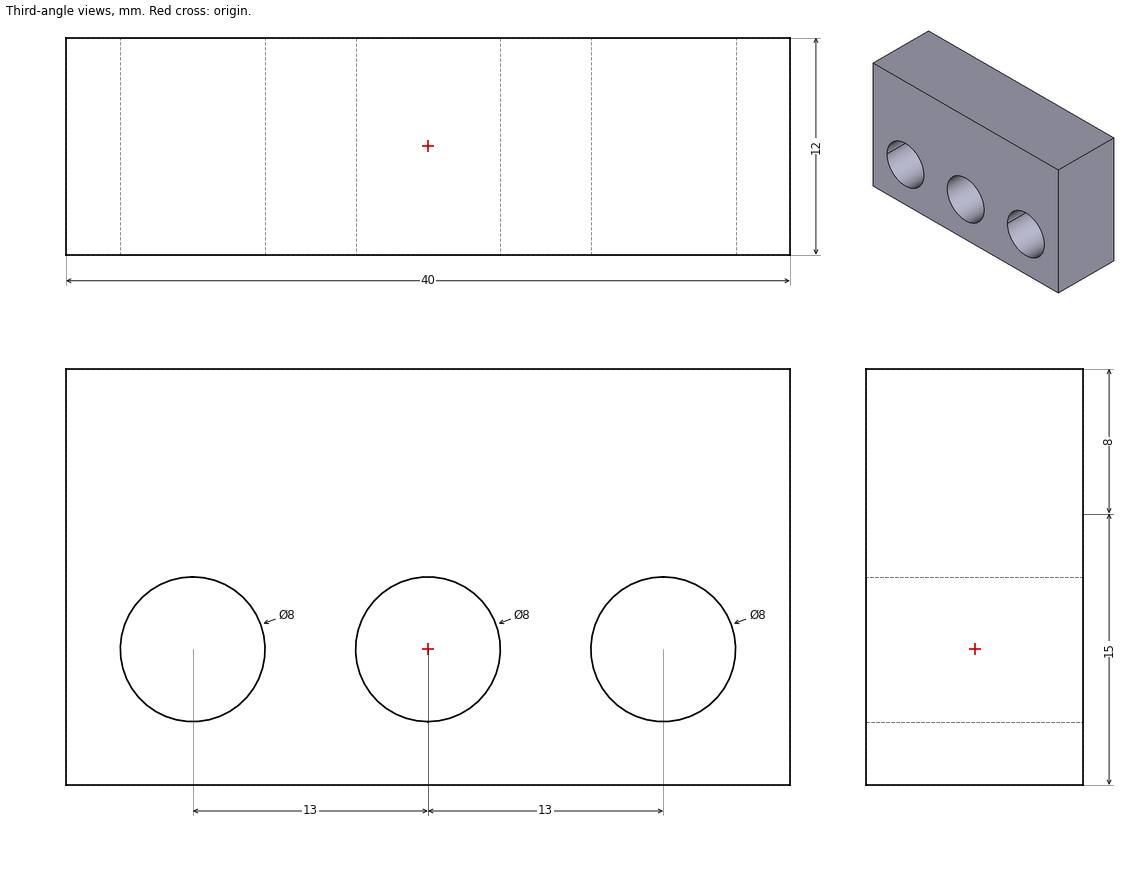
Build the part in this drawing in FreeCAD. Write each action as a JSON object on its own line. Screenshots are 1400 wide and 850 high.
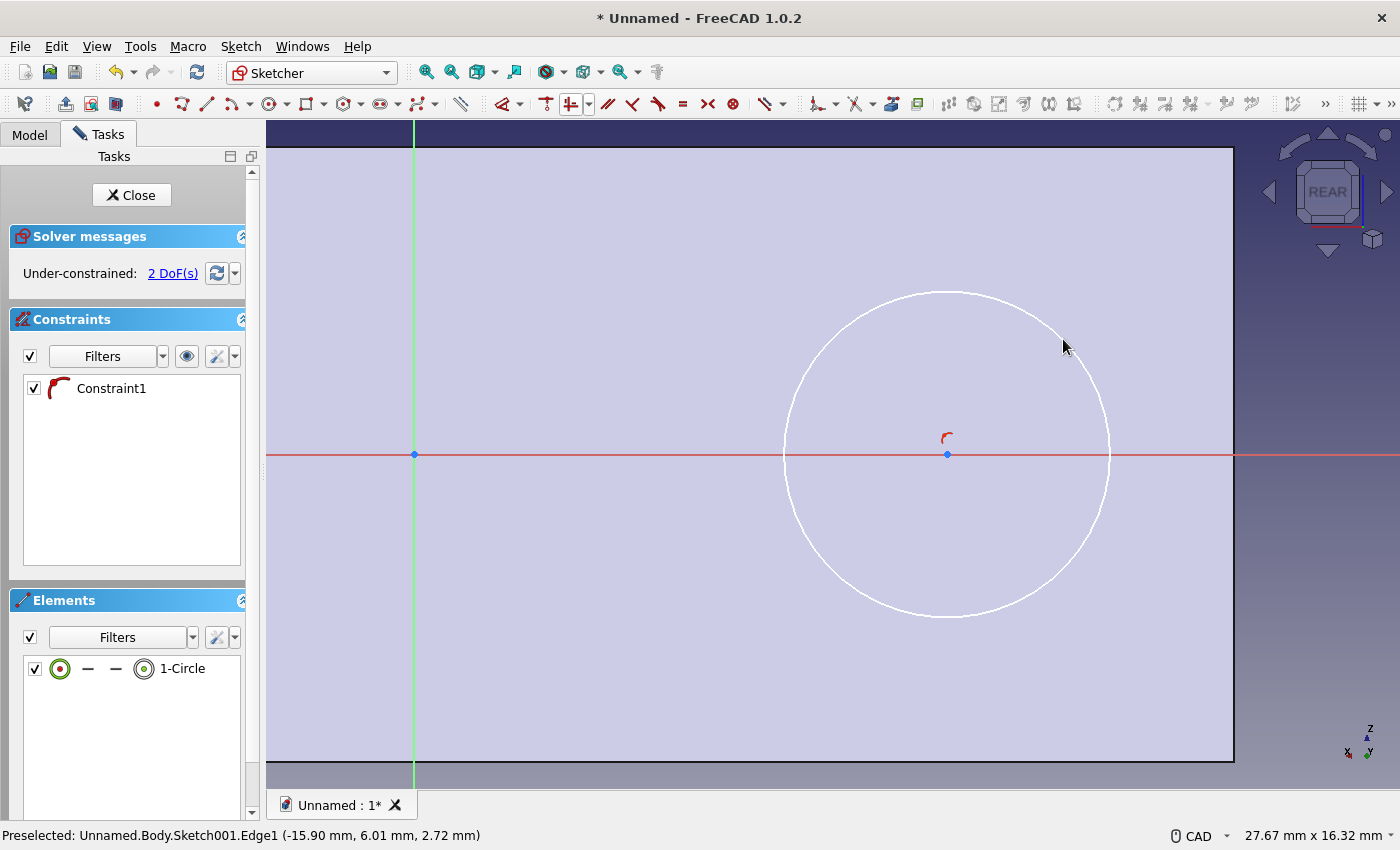
{"action": "key", "text": "d"}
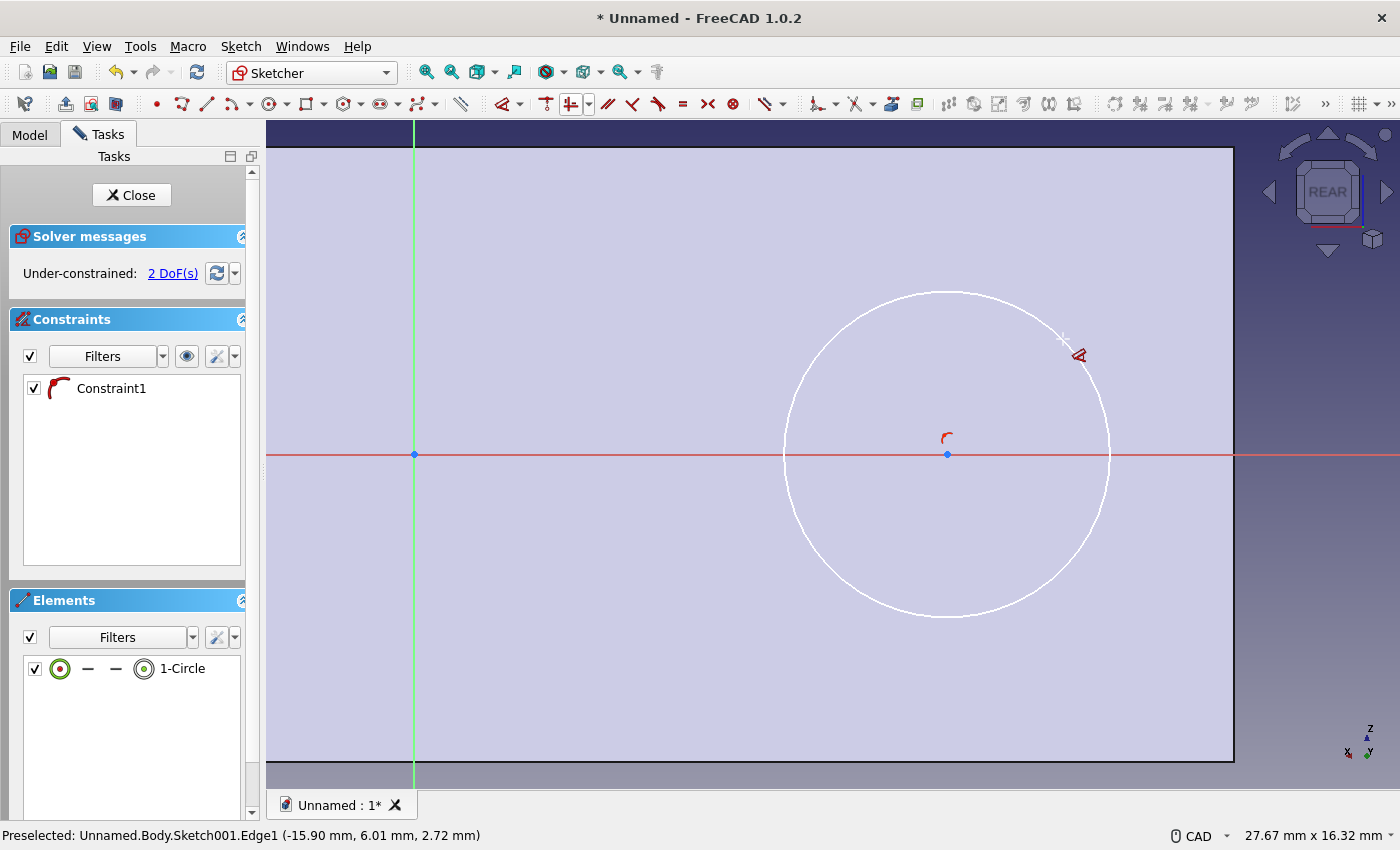
{"action": "left_click", "coordinate": [1062, 339]}
{"action": "left_click", "coordinate": [1085, 316]}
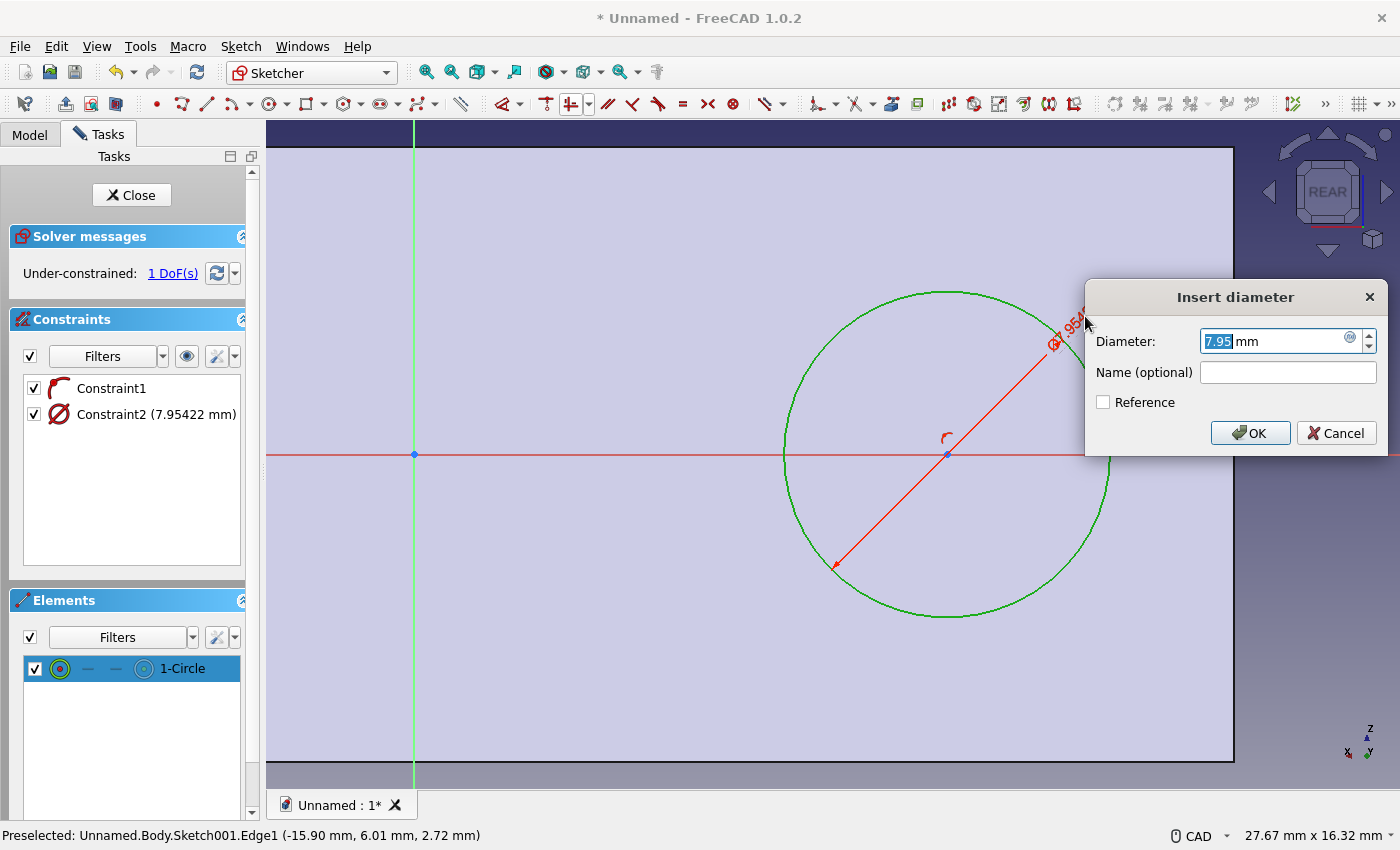
{"action": "type", "text": "8"}
{"action": "key", "text": "Return"}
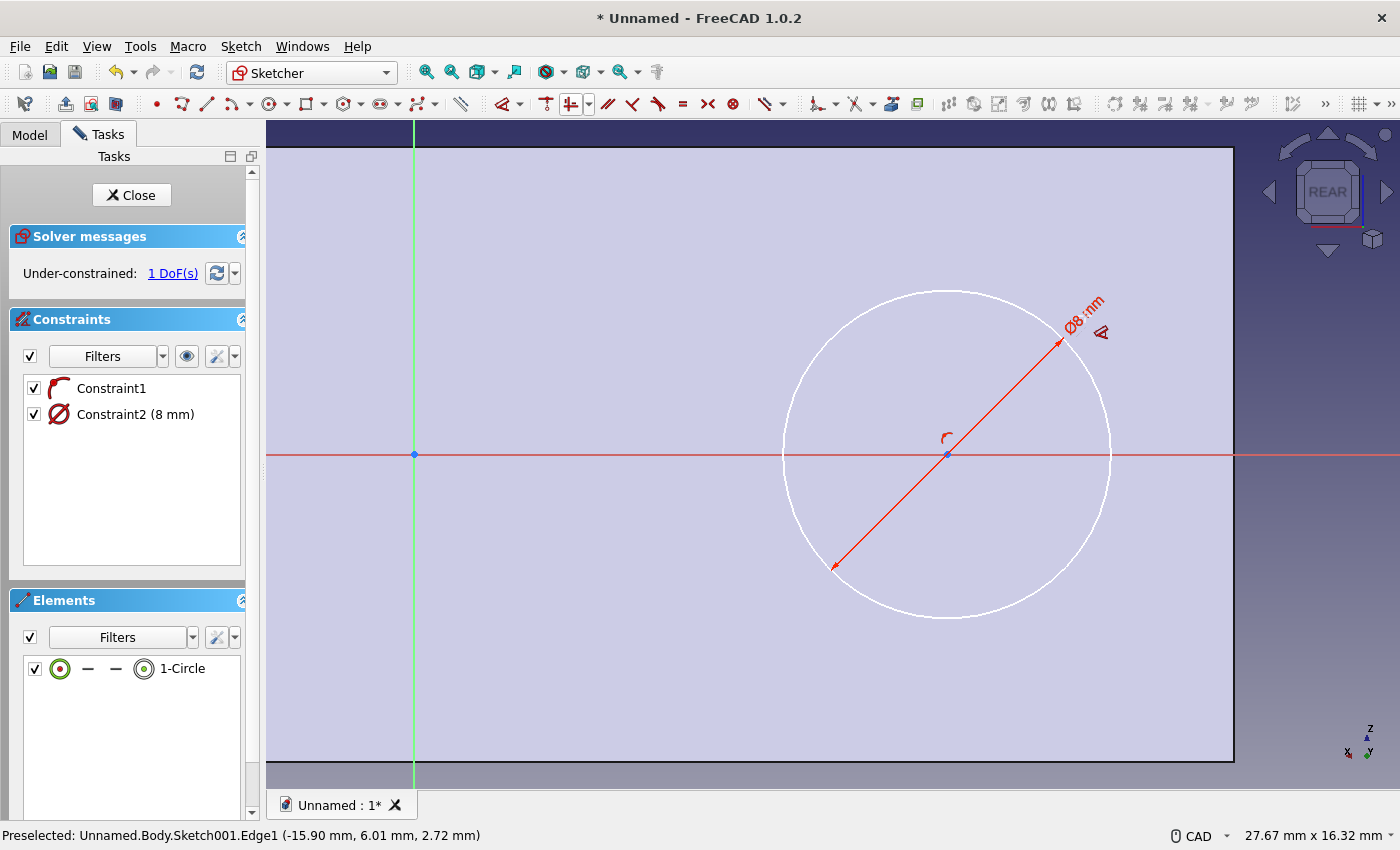
{"action": "left_click", "coordinate": [947, 454]}
{"action": "left_click", "coordinate": [681, 488]}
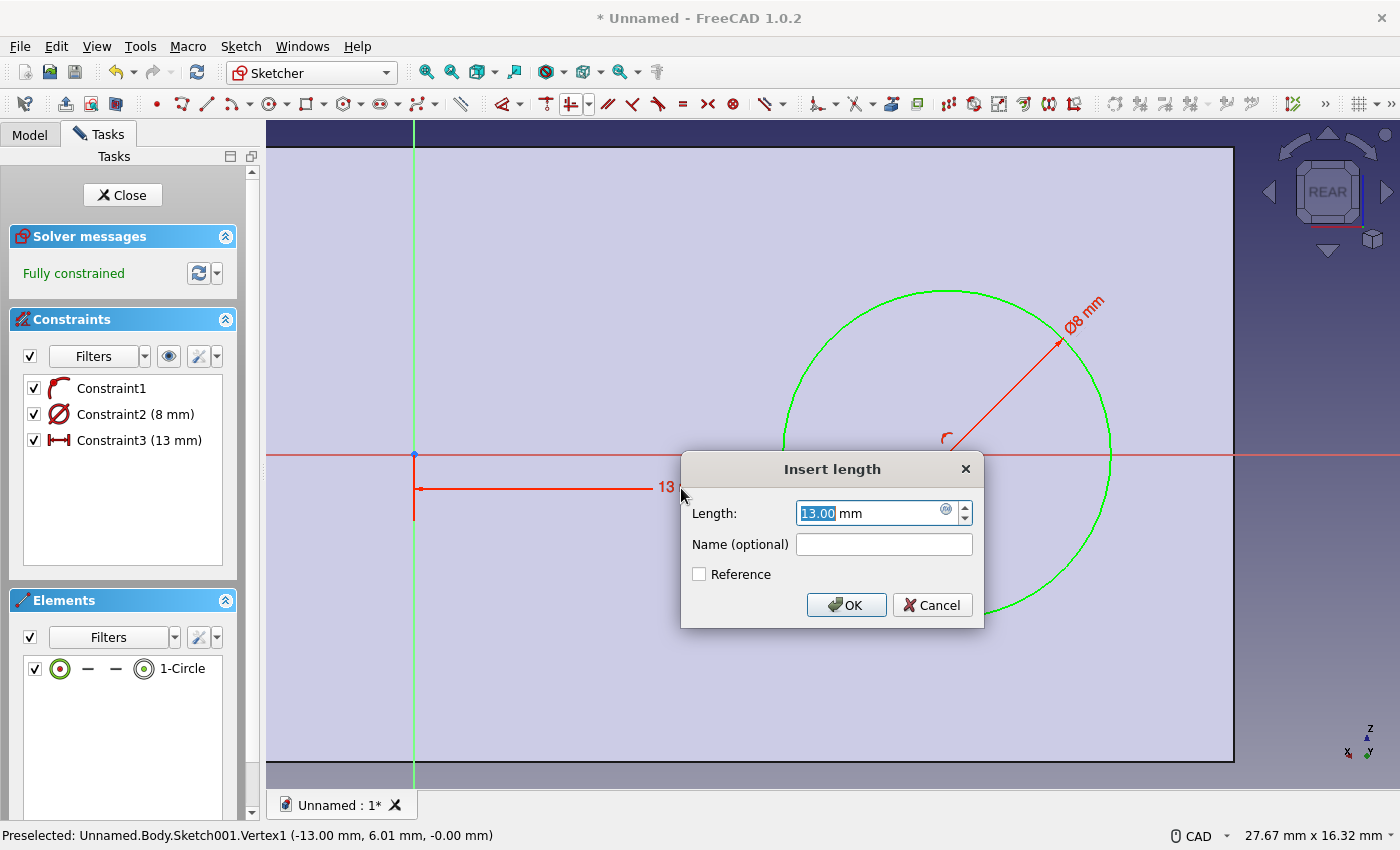
{"action": "type", "text": "13"}
{"action": "key", "text": "Return"}
{"action": "key", "text": "Escape"}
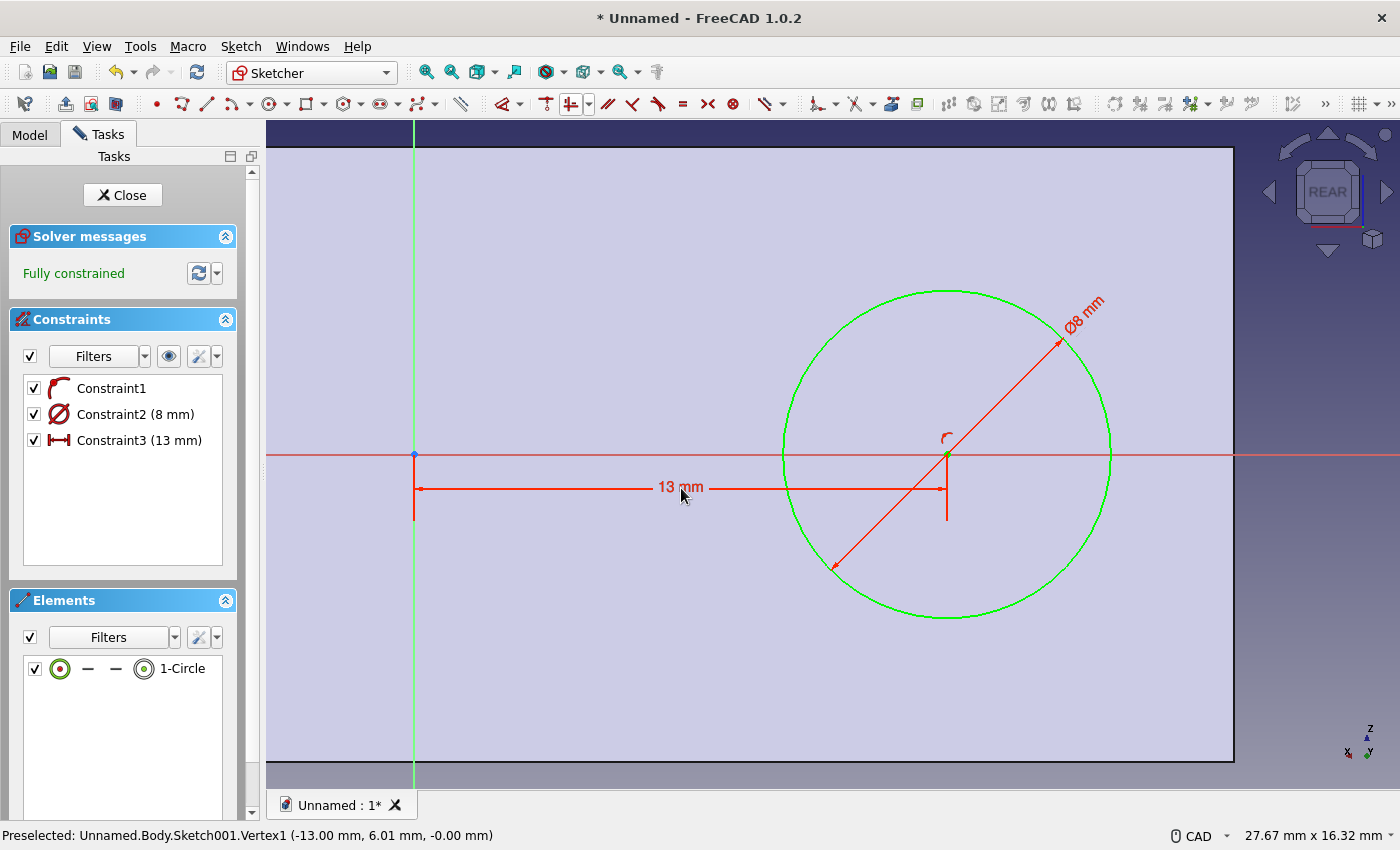
{"action": "left_click", "coordinate": [123, 195]}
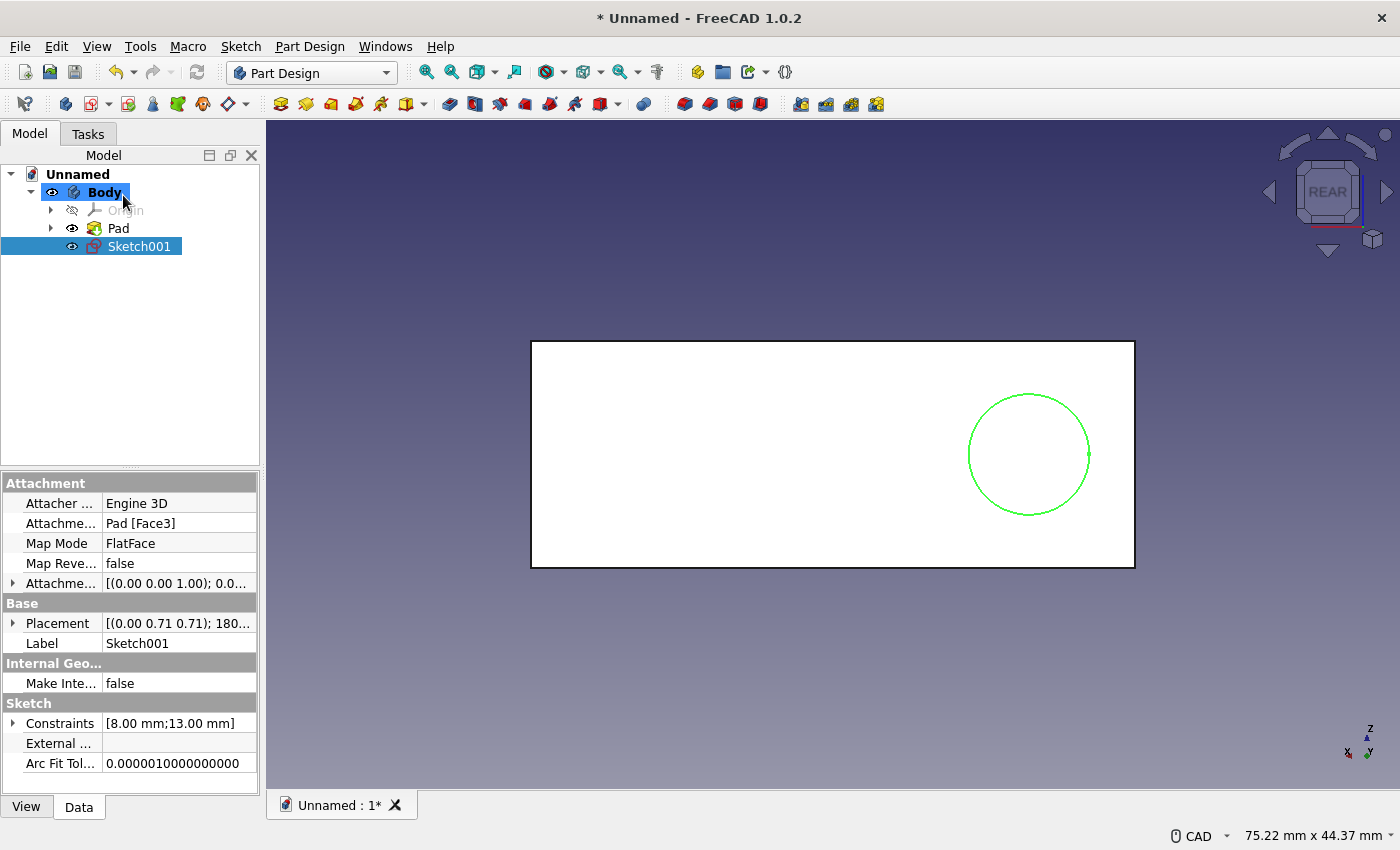
{"action": "left_click", "coordinate": [450, 104]}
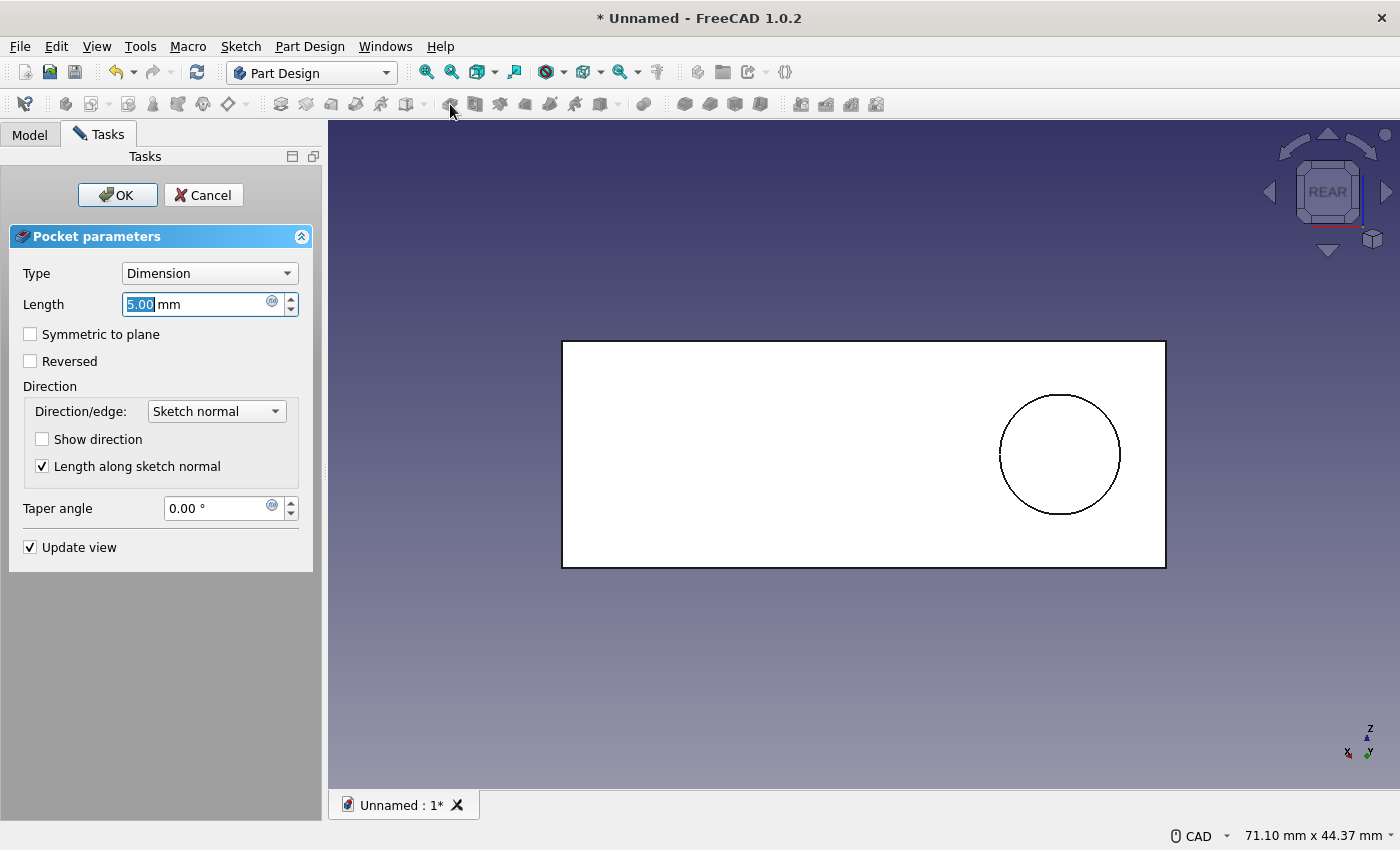
{"action": "left_click", "coordinate": [210, 274]}